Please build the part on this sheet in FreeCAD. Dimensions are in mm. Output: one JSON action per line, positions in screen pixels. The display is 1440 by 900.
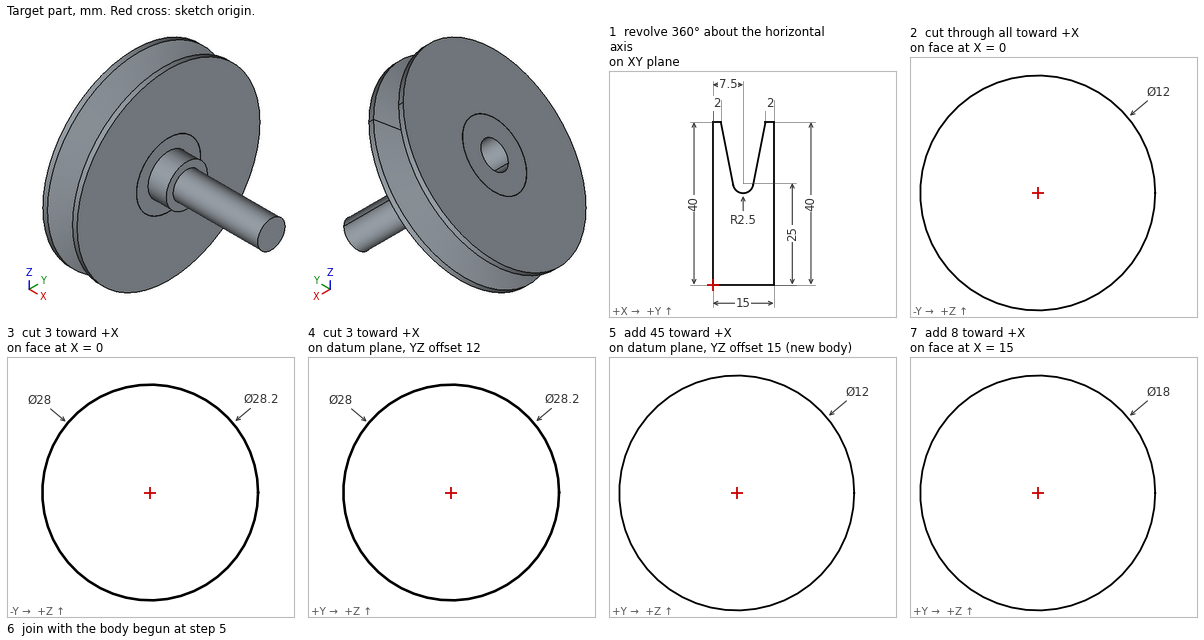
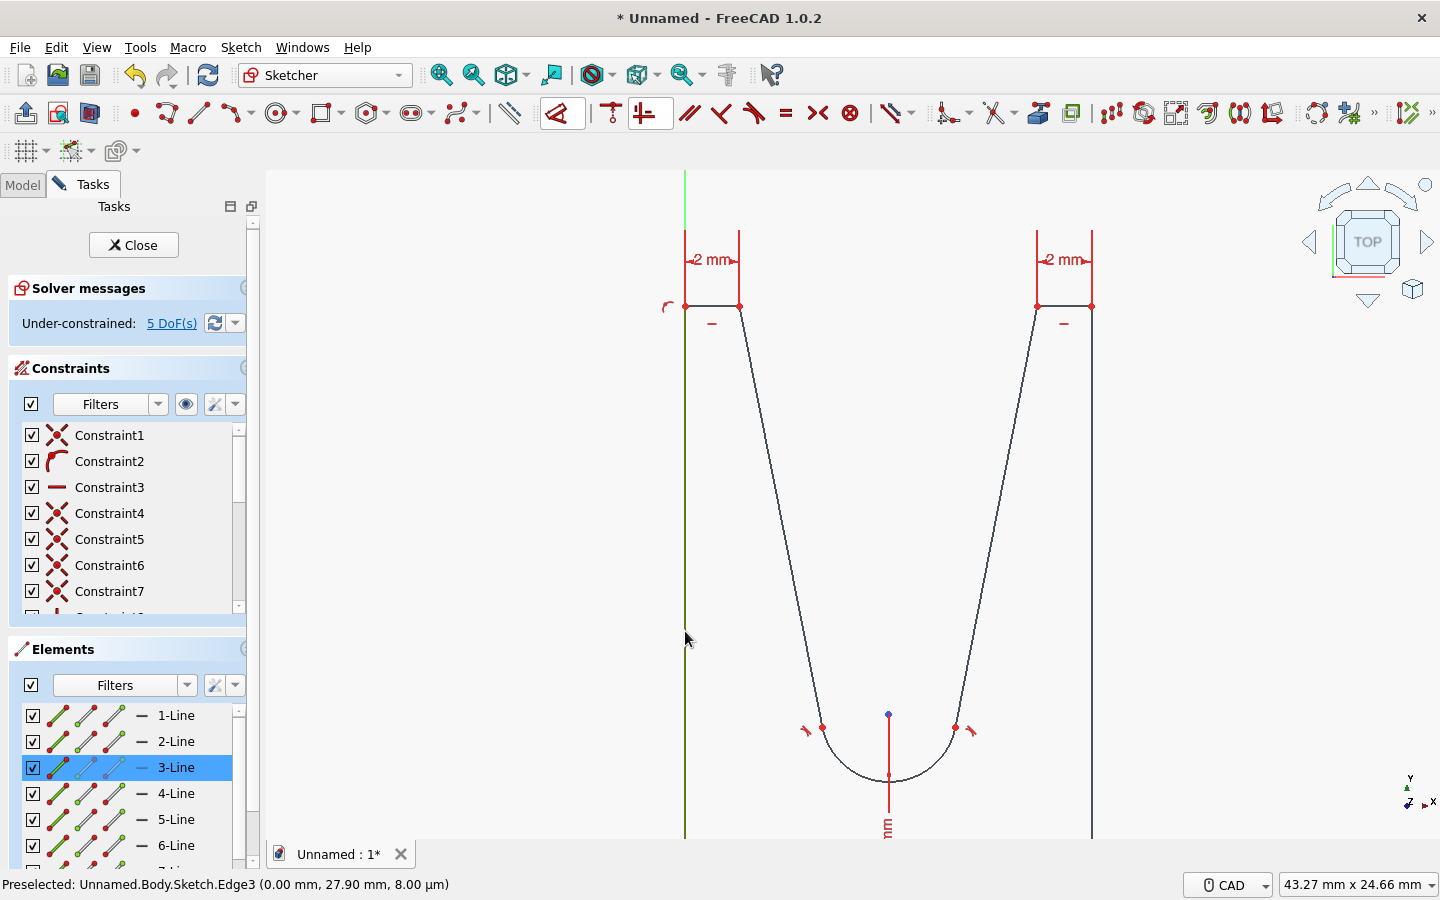
{"action": "key", "text": "i"}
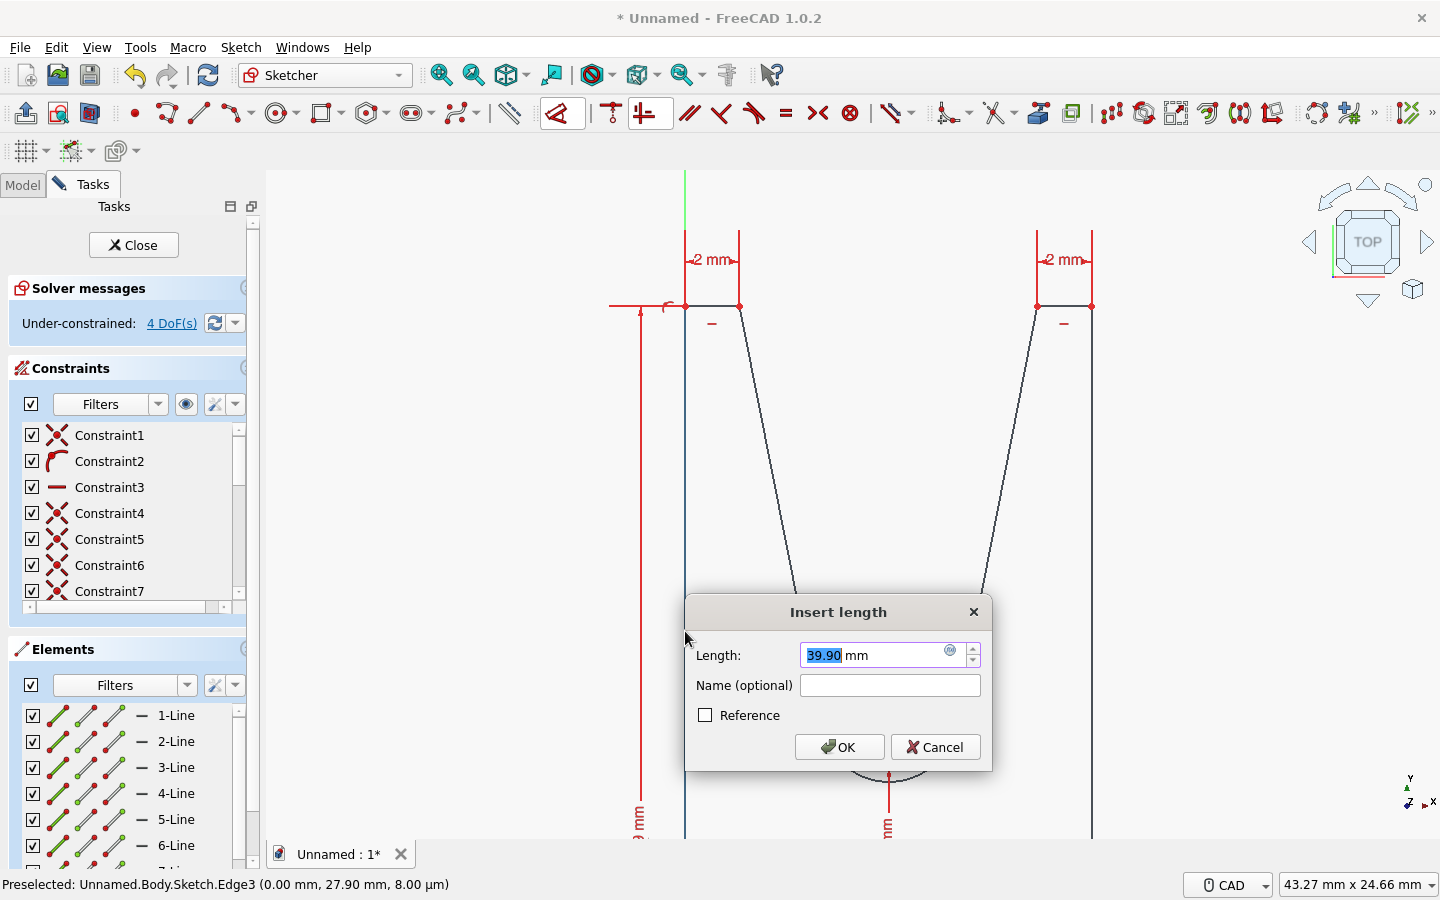
{"action": "type", "text": "40"}
{"action": "key", "text": "Return"}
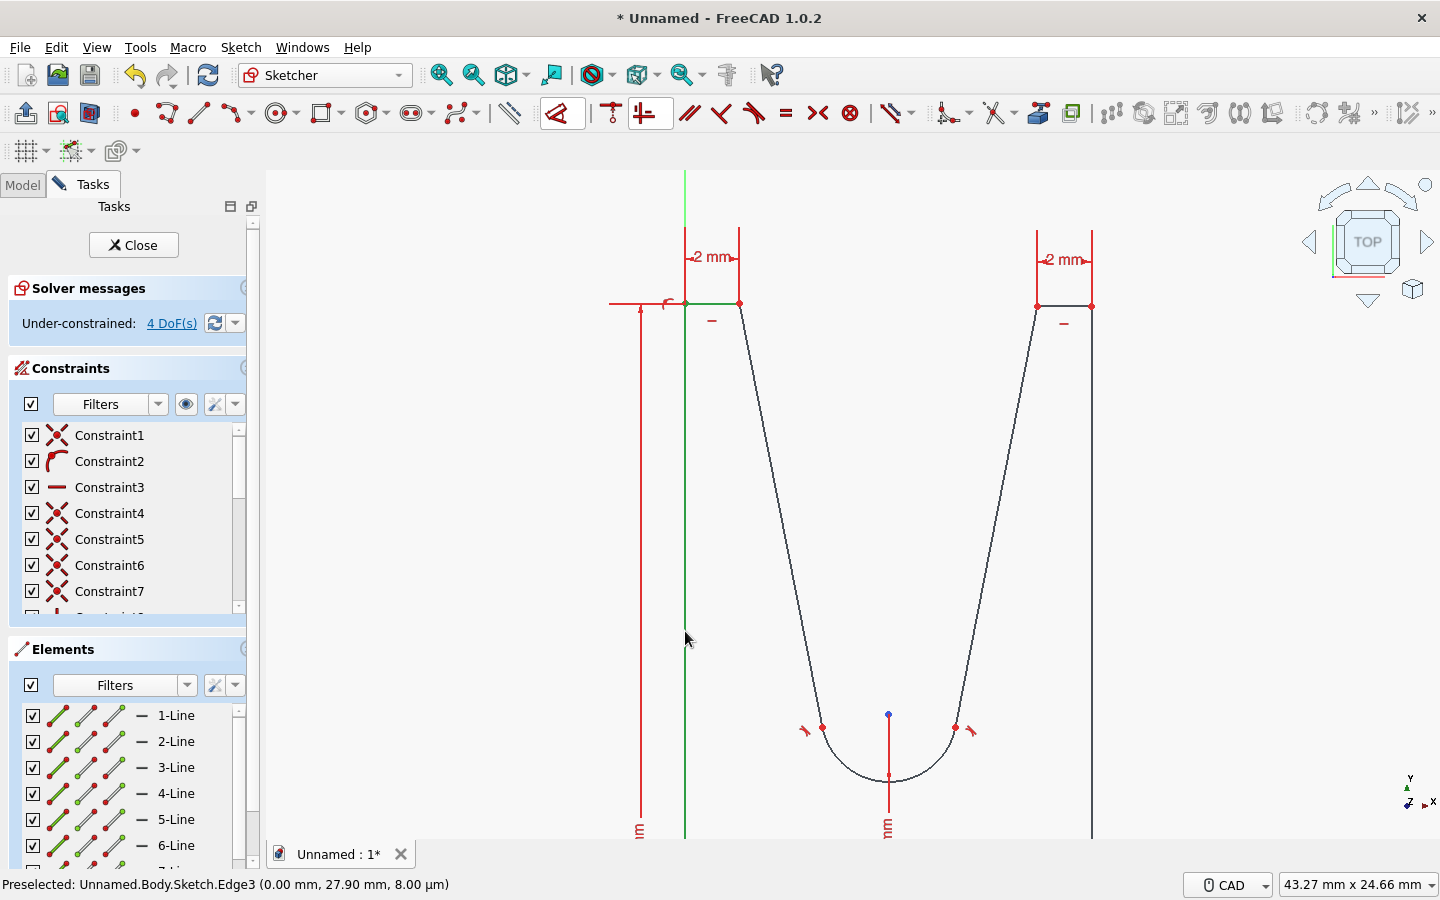
{"action": "scroll", "coordinate": [724, 306], "scroll_direction": "down", "scroll_amount": 5}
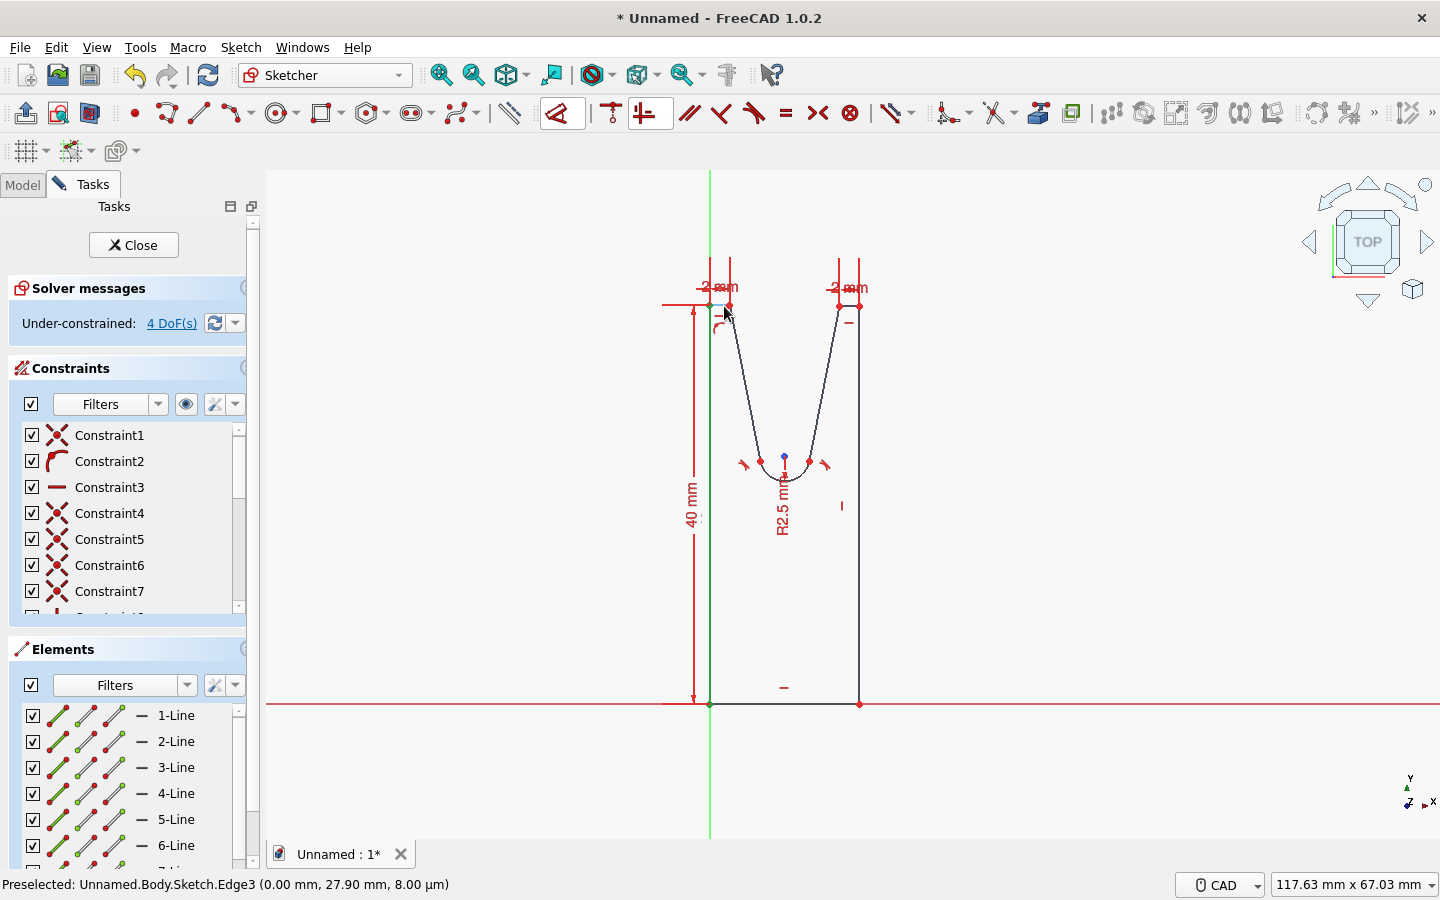
{"action": "left_click", "coordinate": [755, 704]}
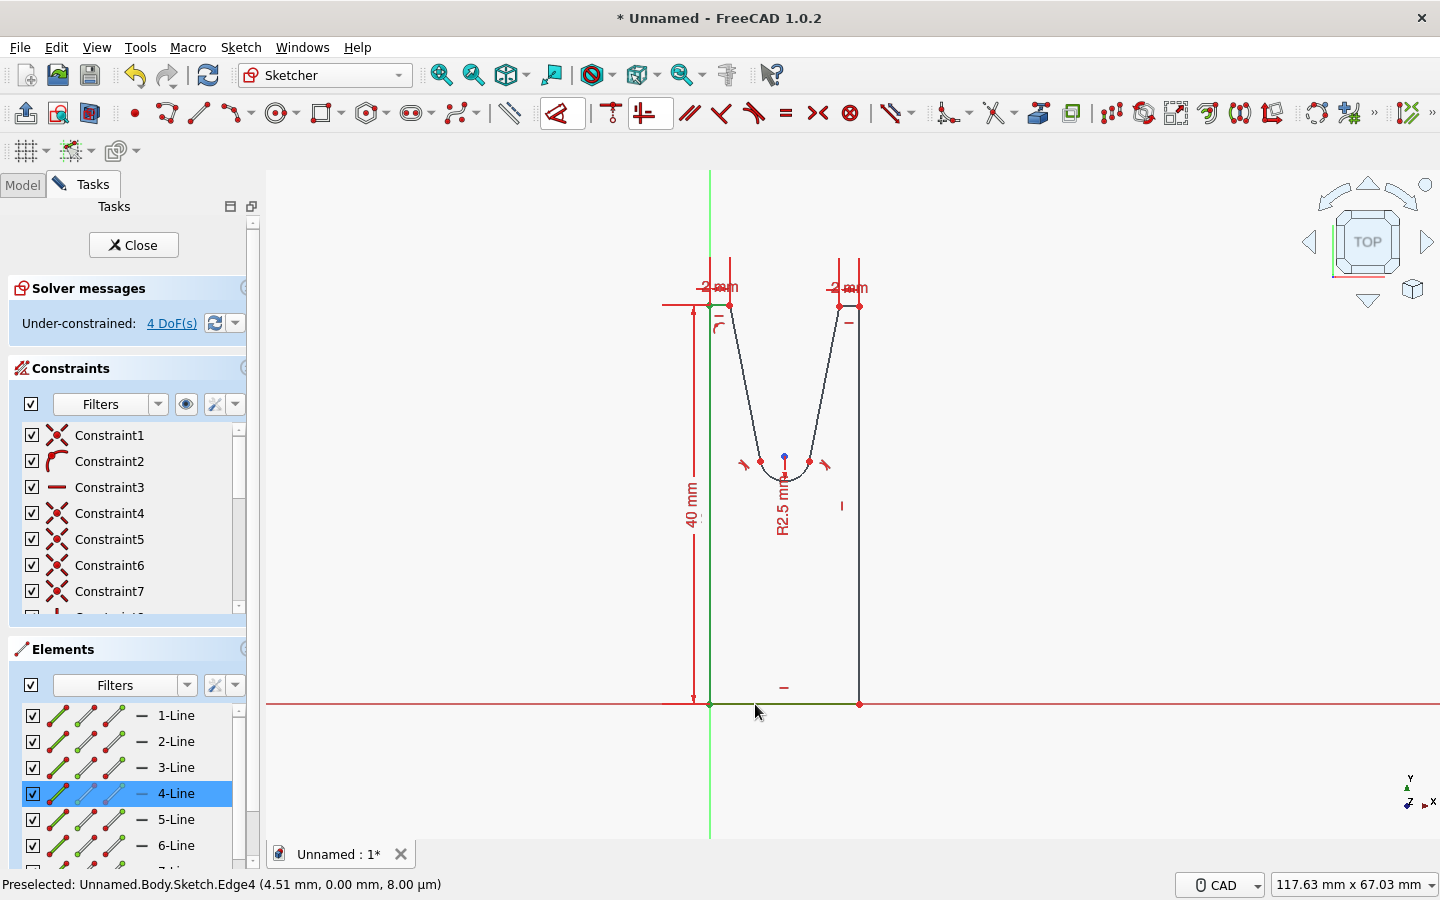
{"action": "key", "text": "l"}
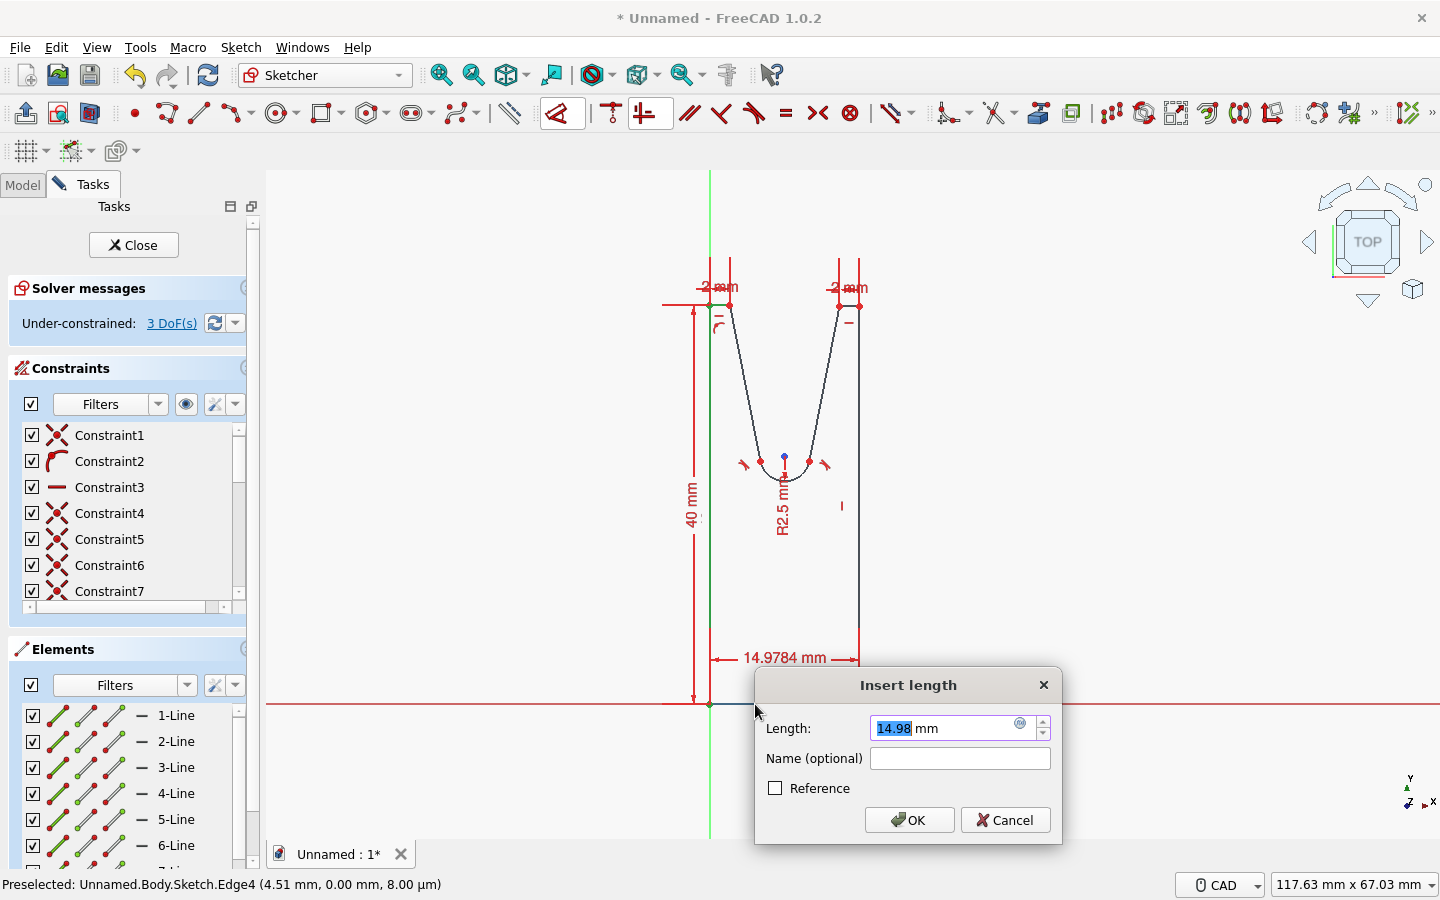
{"action": "type", "text": "15"}
{"action": "key", "text": "Return"}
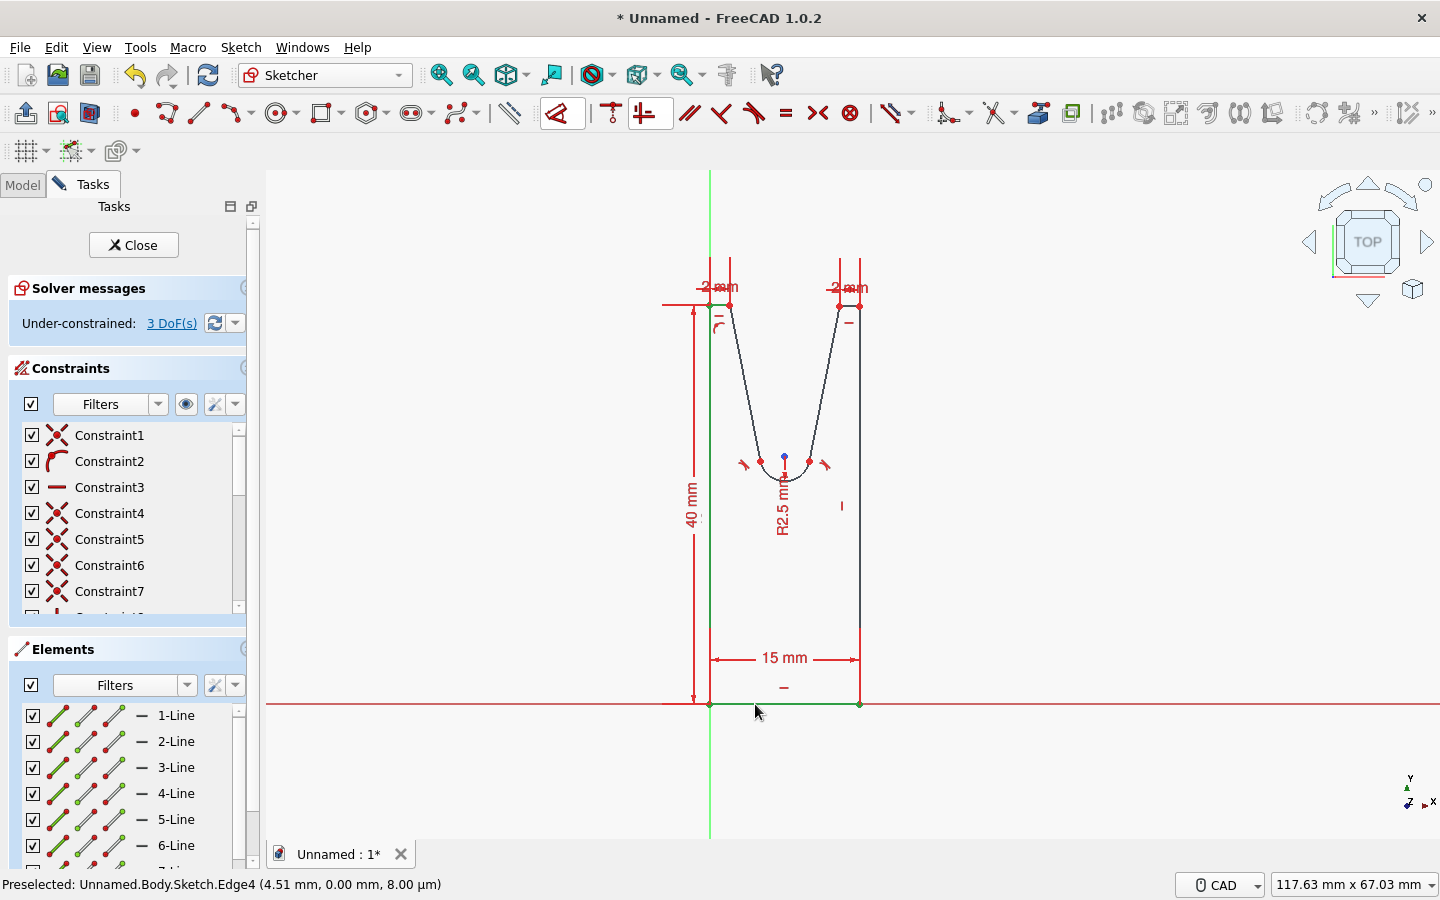
{"action": "left_click", "coordinate": [860, 585]}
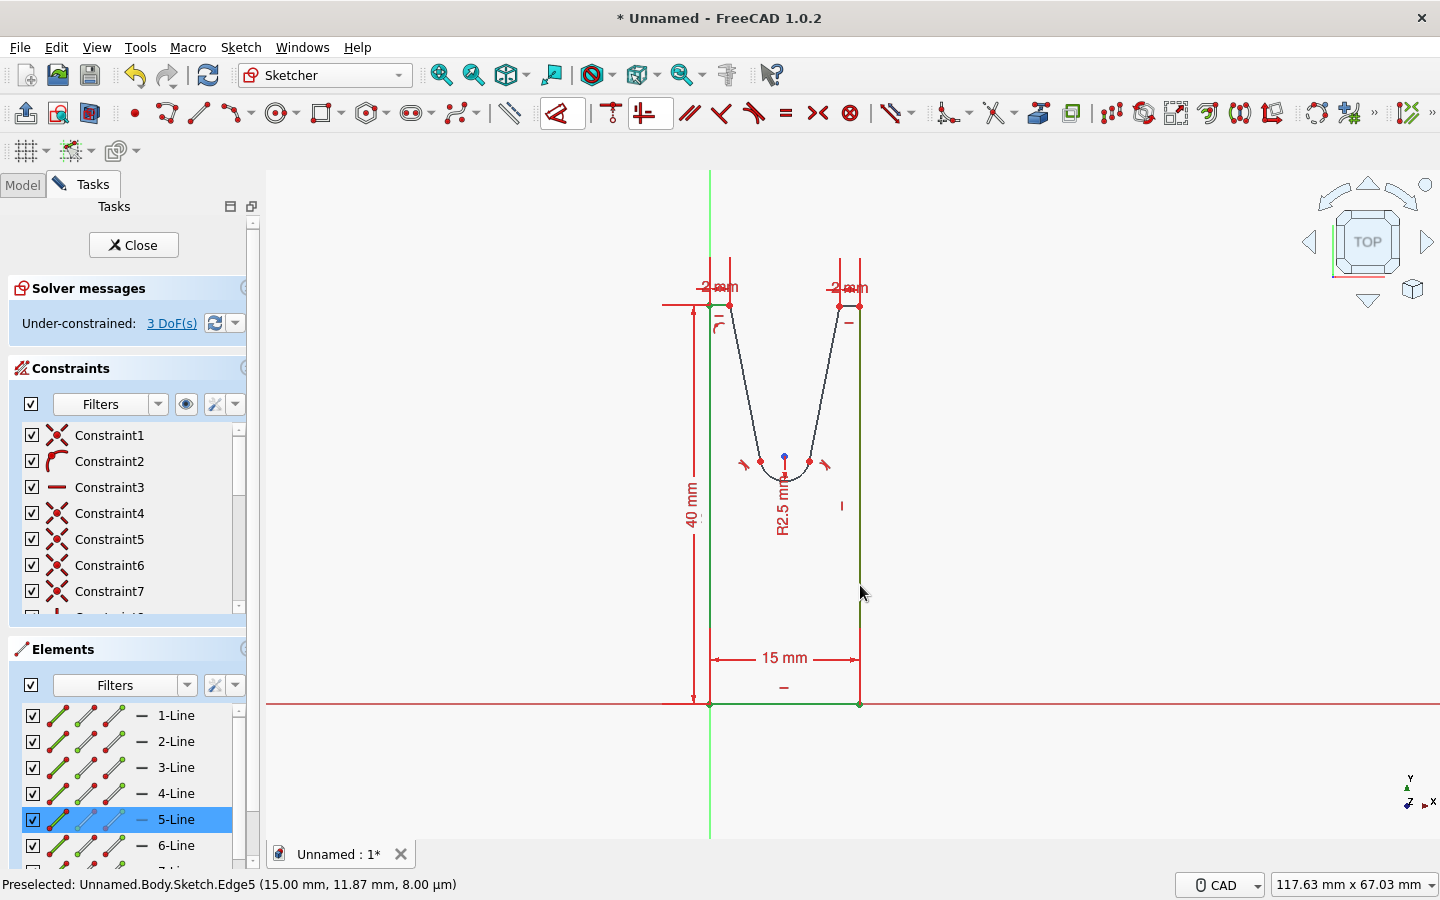
{"action": "left_click", "coordinate": [580, 114]}